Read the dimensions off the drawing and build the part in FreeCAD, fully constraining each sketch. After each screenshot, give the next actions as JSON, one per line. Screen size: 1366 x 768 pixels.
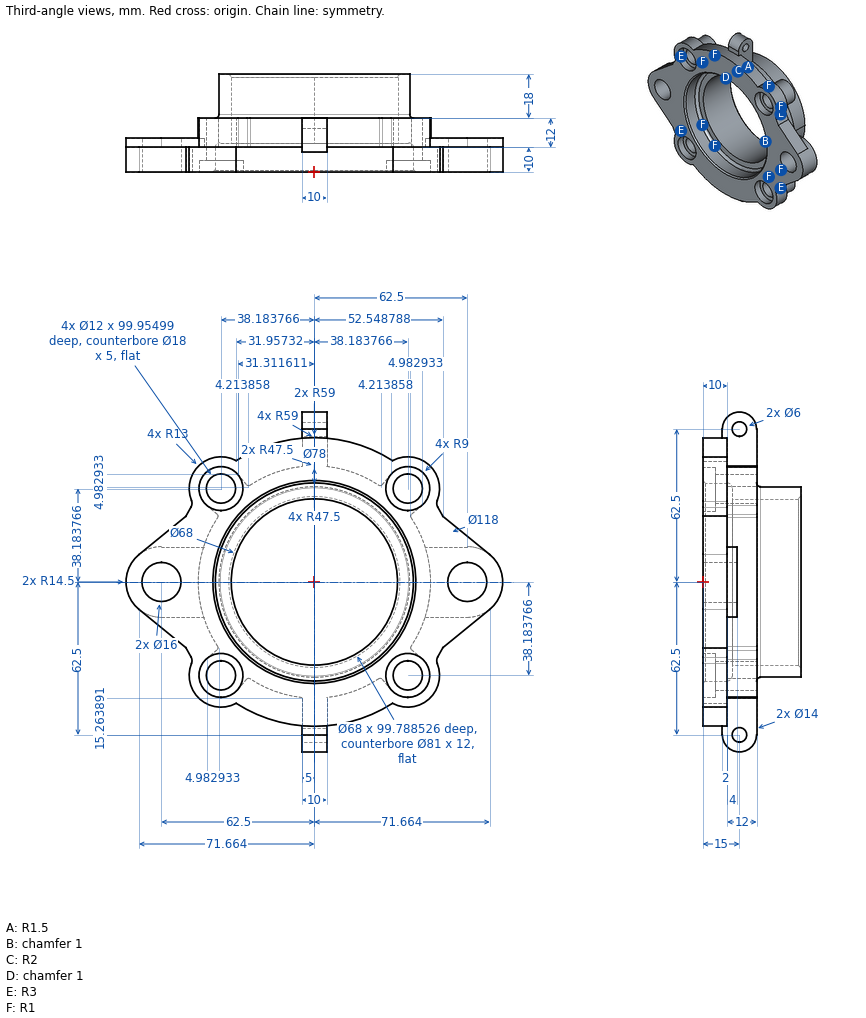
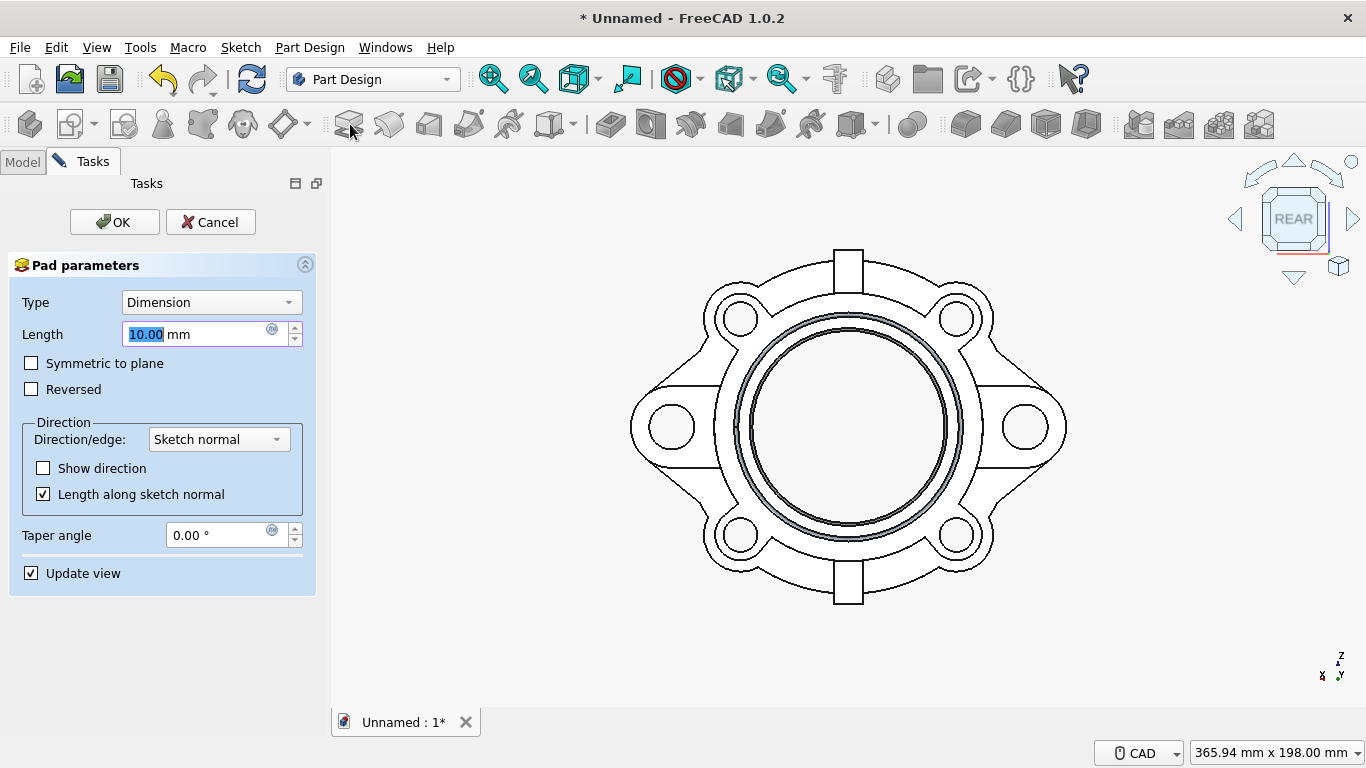
{"action": "left_click", "coordinate": [212, 302]}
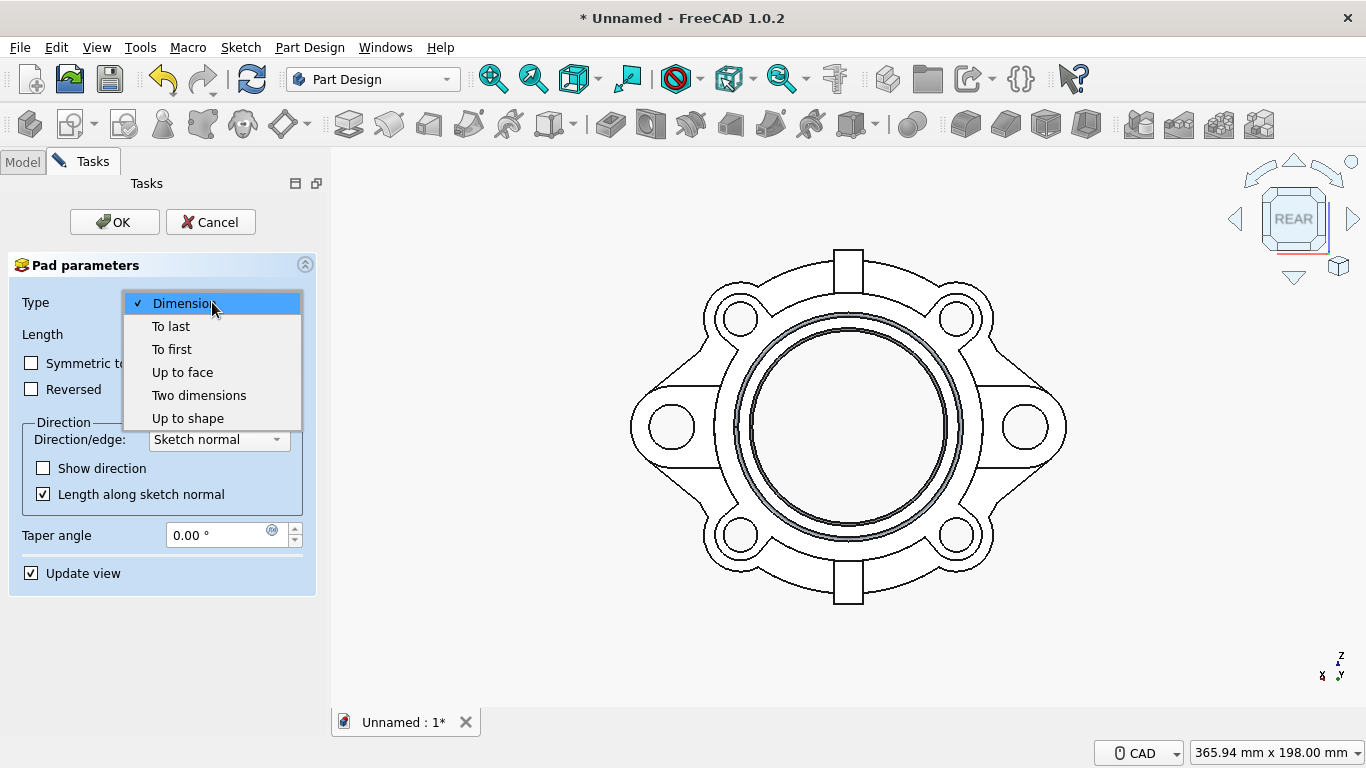
{"action": "left_click", "coordinate": [212, 396]}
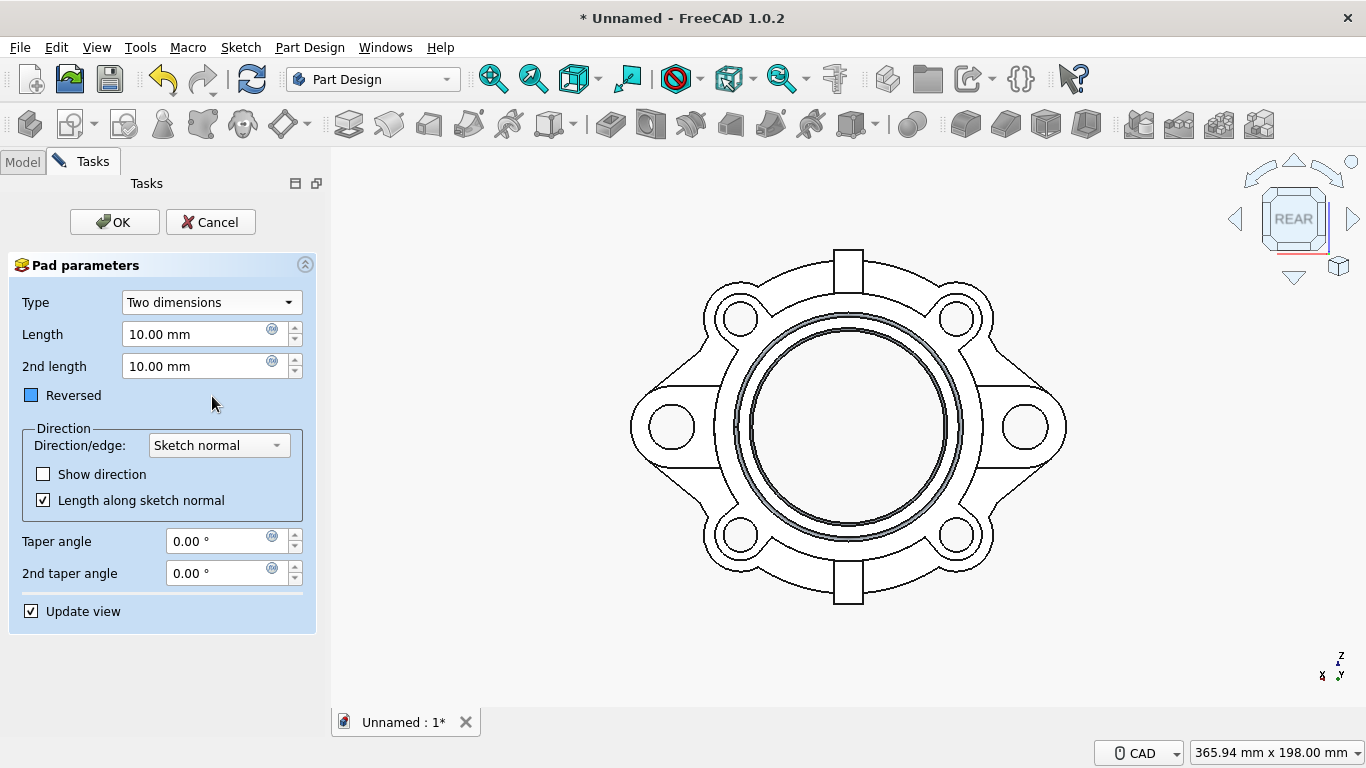
{"action": "triple_click", "coordinate": [204, 334]}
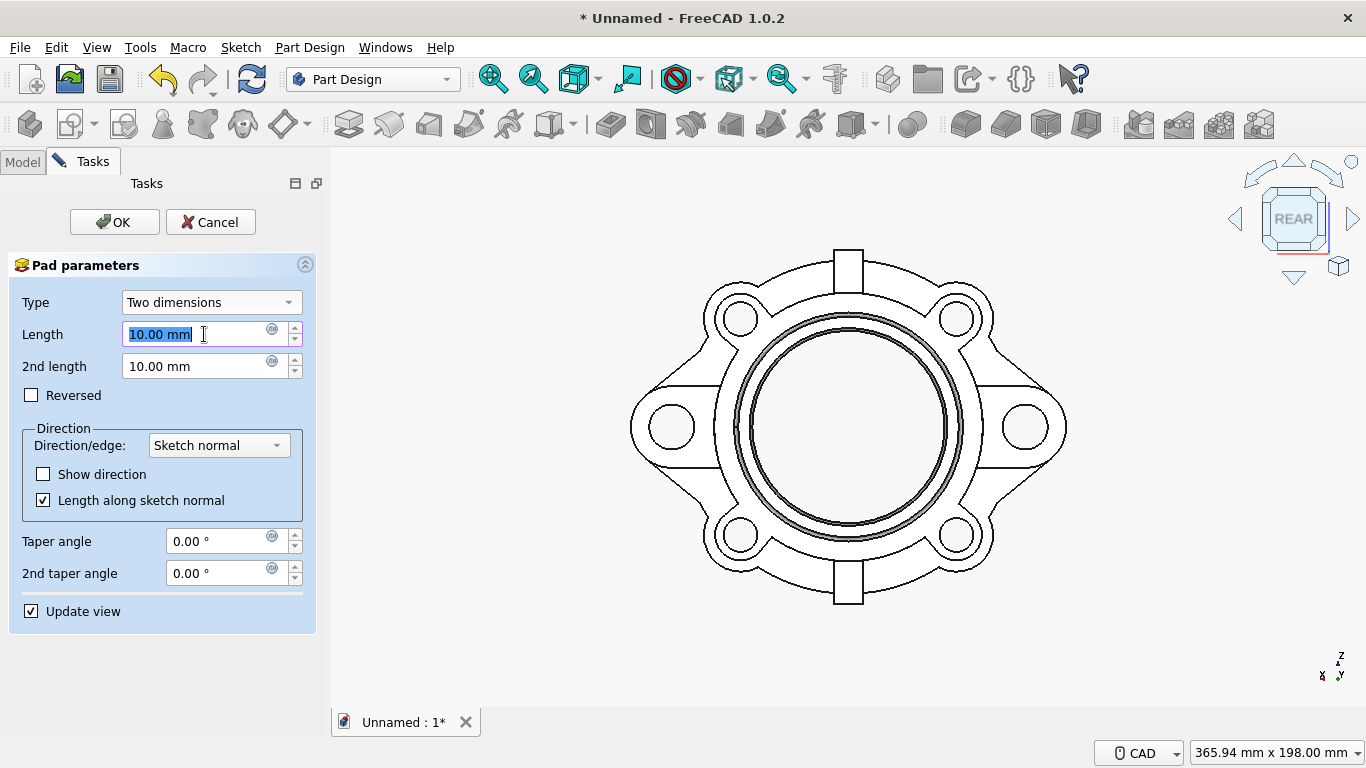
{"action": "type", "text": "12"}
{"action": "key", "text": "Tab"}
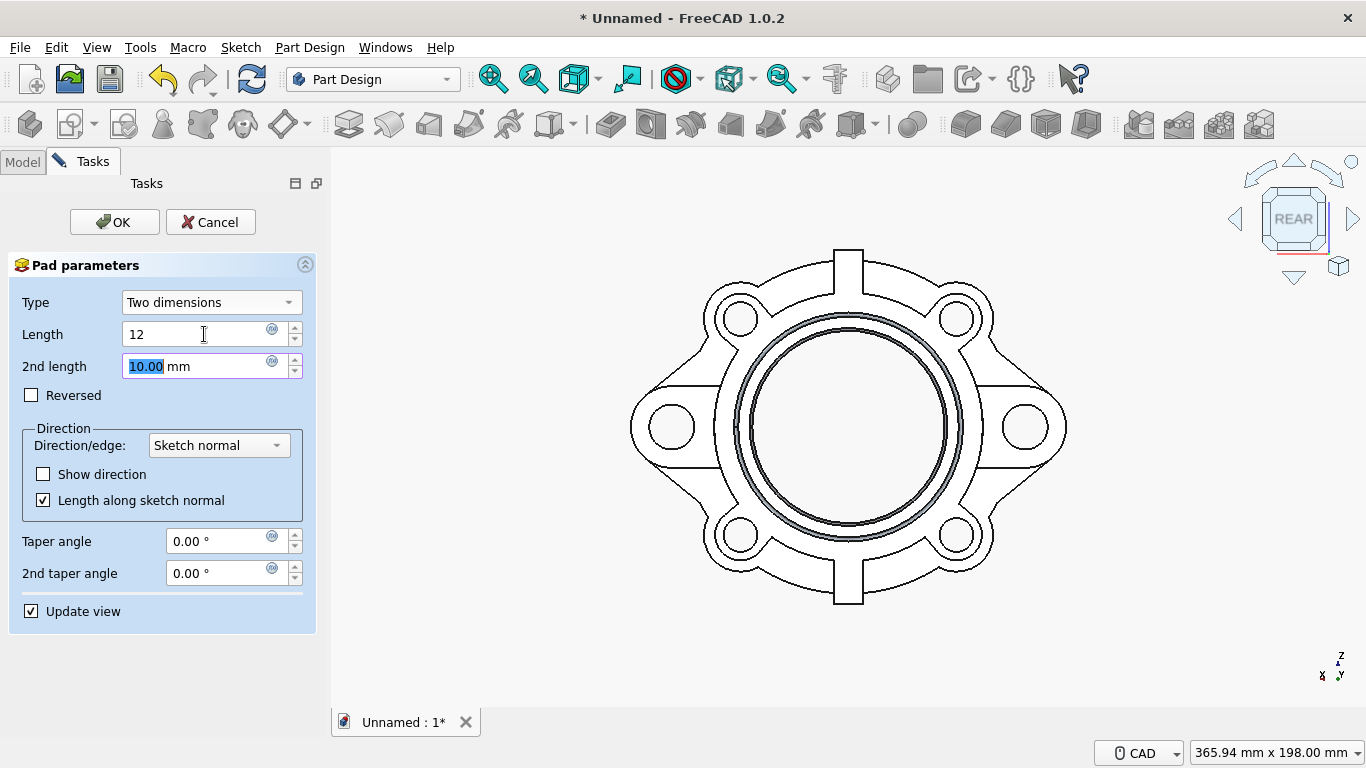
{"action": "type", "text": "2"}
{"action": "key", "text": "Tab"}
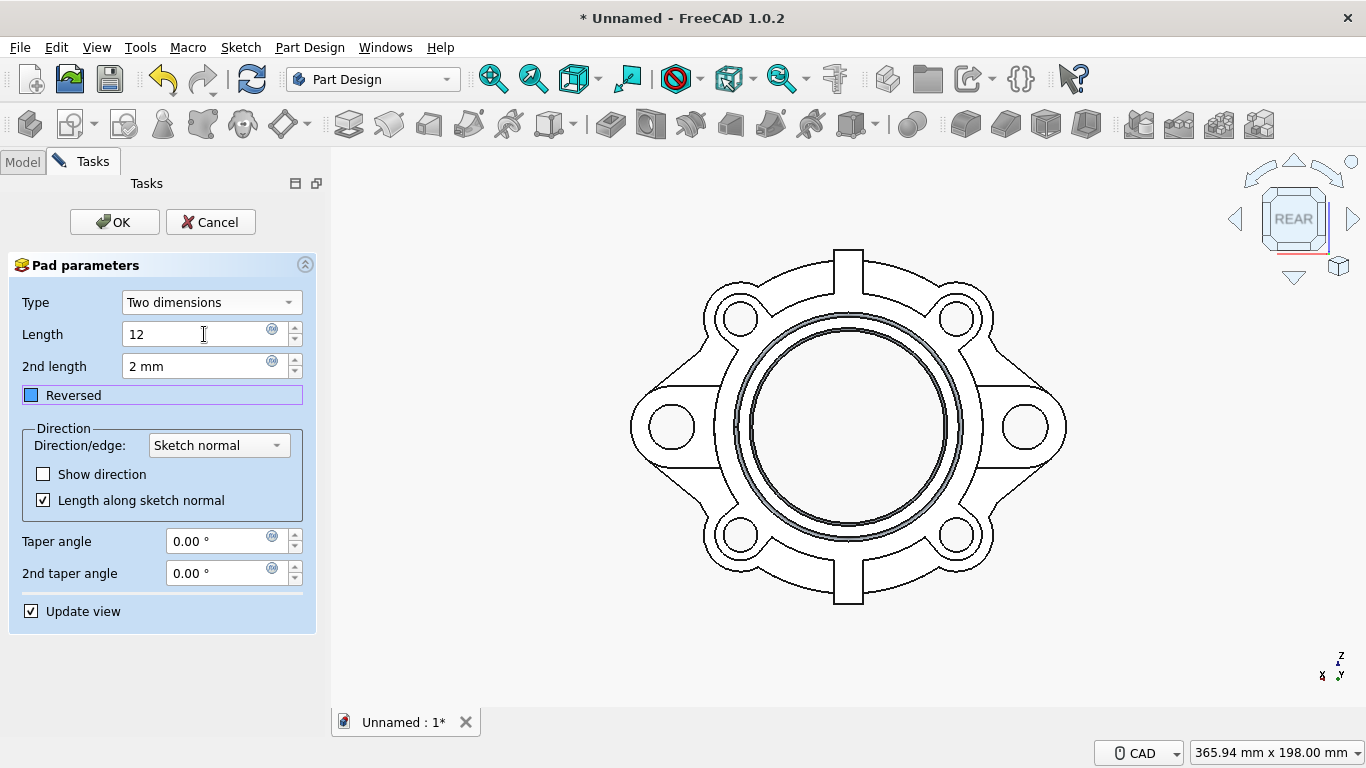
{"action": "left_click", "coordinate": [115, 222]}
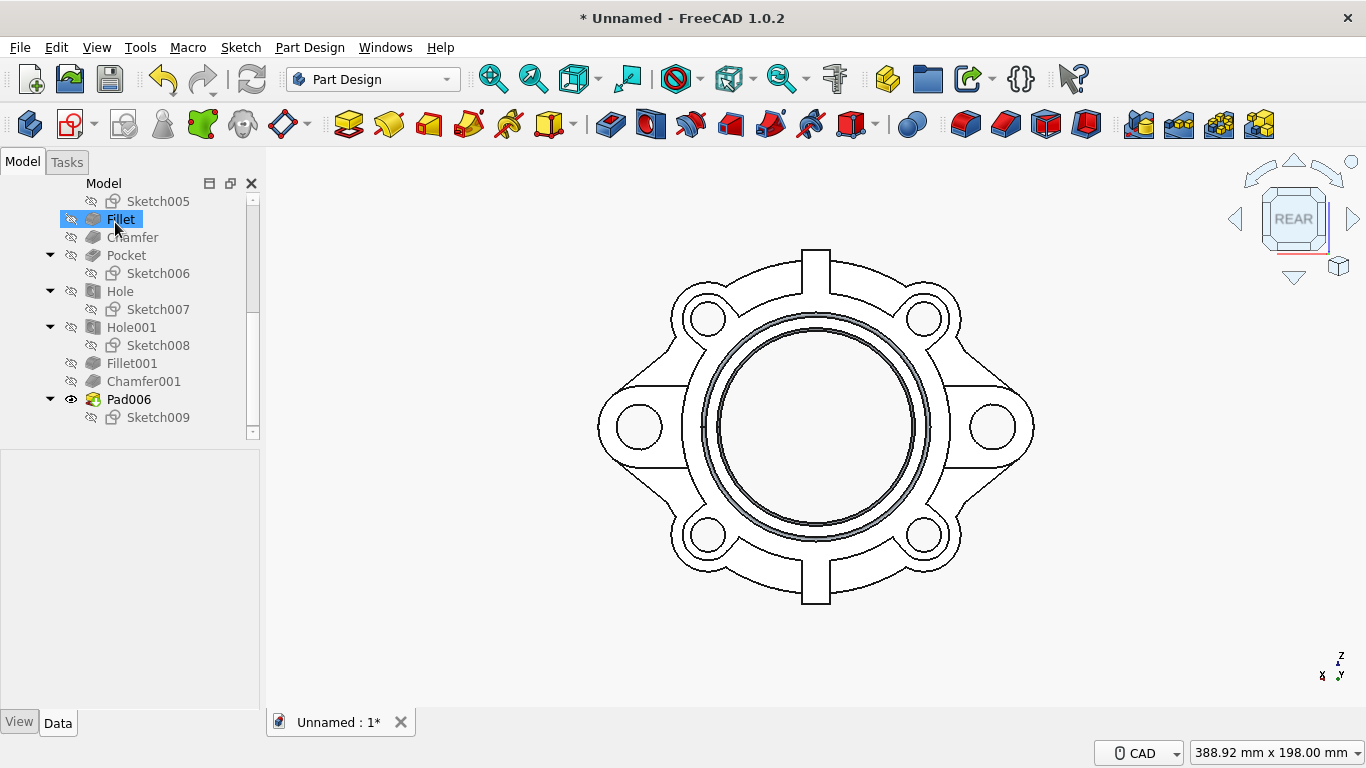
{"action": "key", "text": "0"}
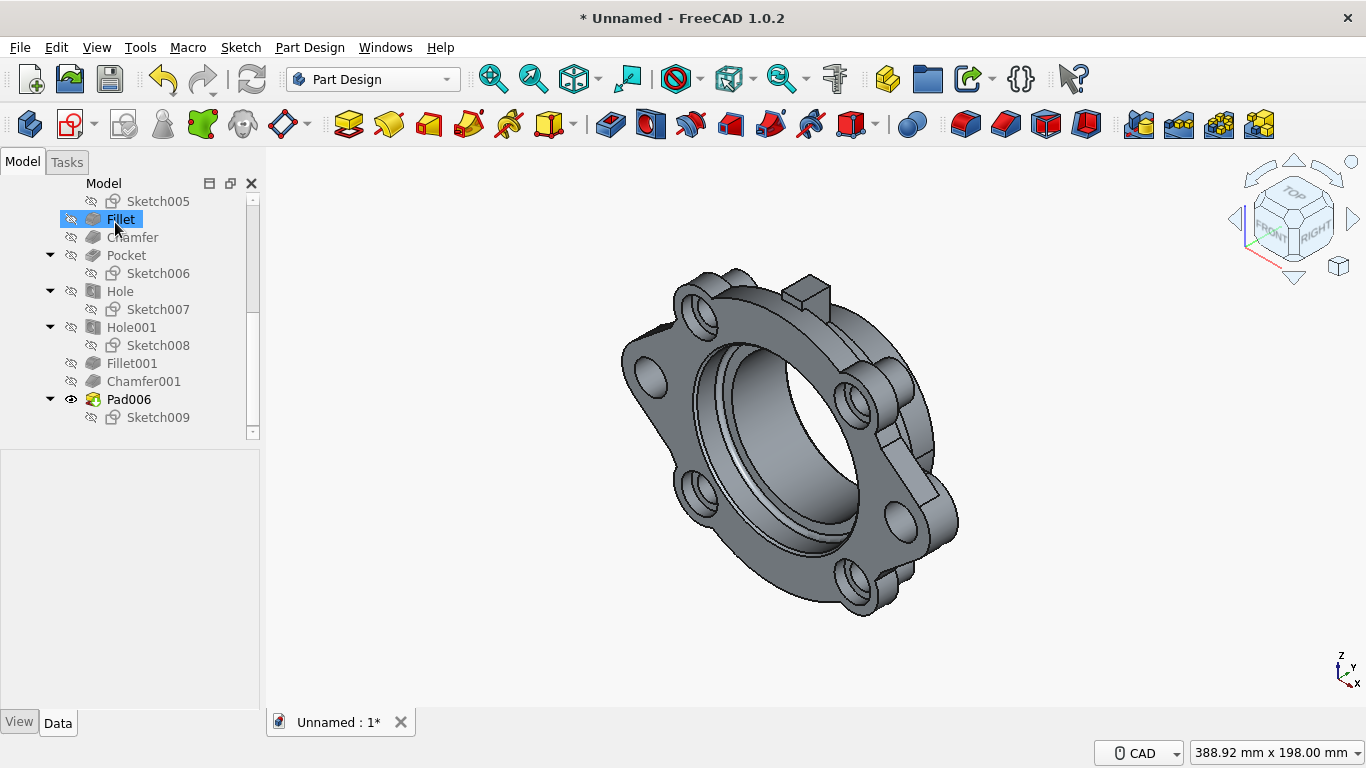
{"action": "key", "text": "3"}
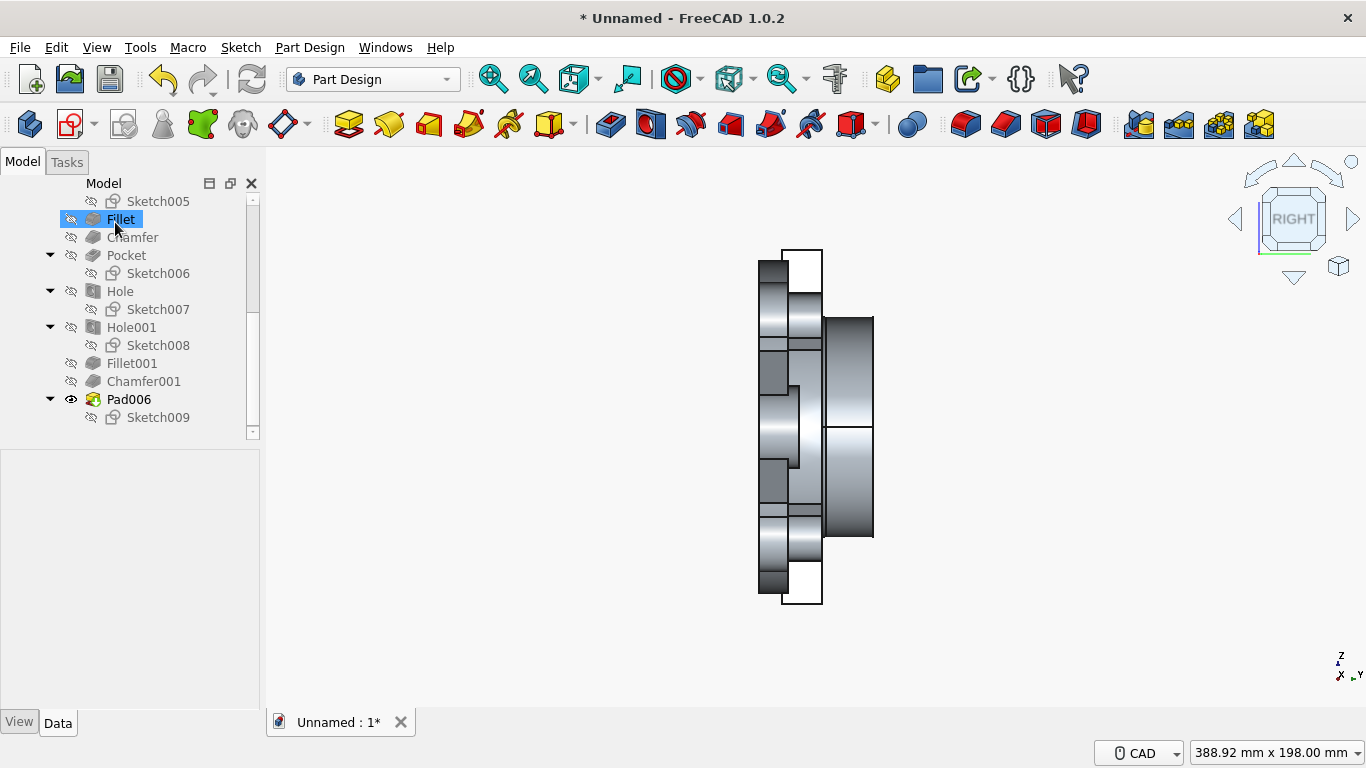
{"action": "left_click", "coordinate": [802, 575]}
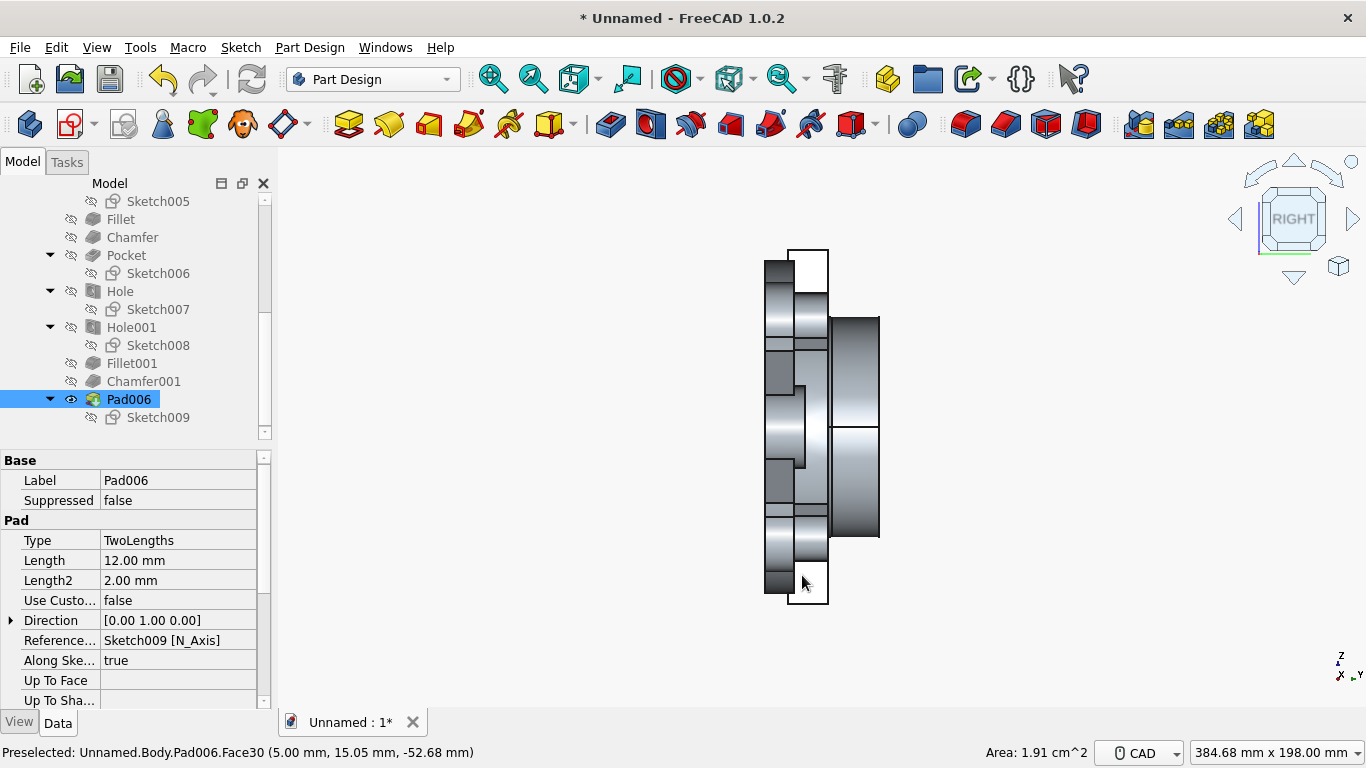
{"action": "left_click", "coordinate": [70, 124]}